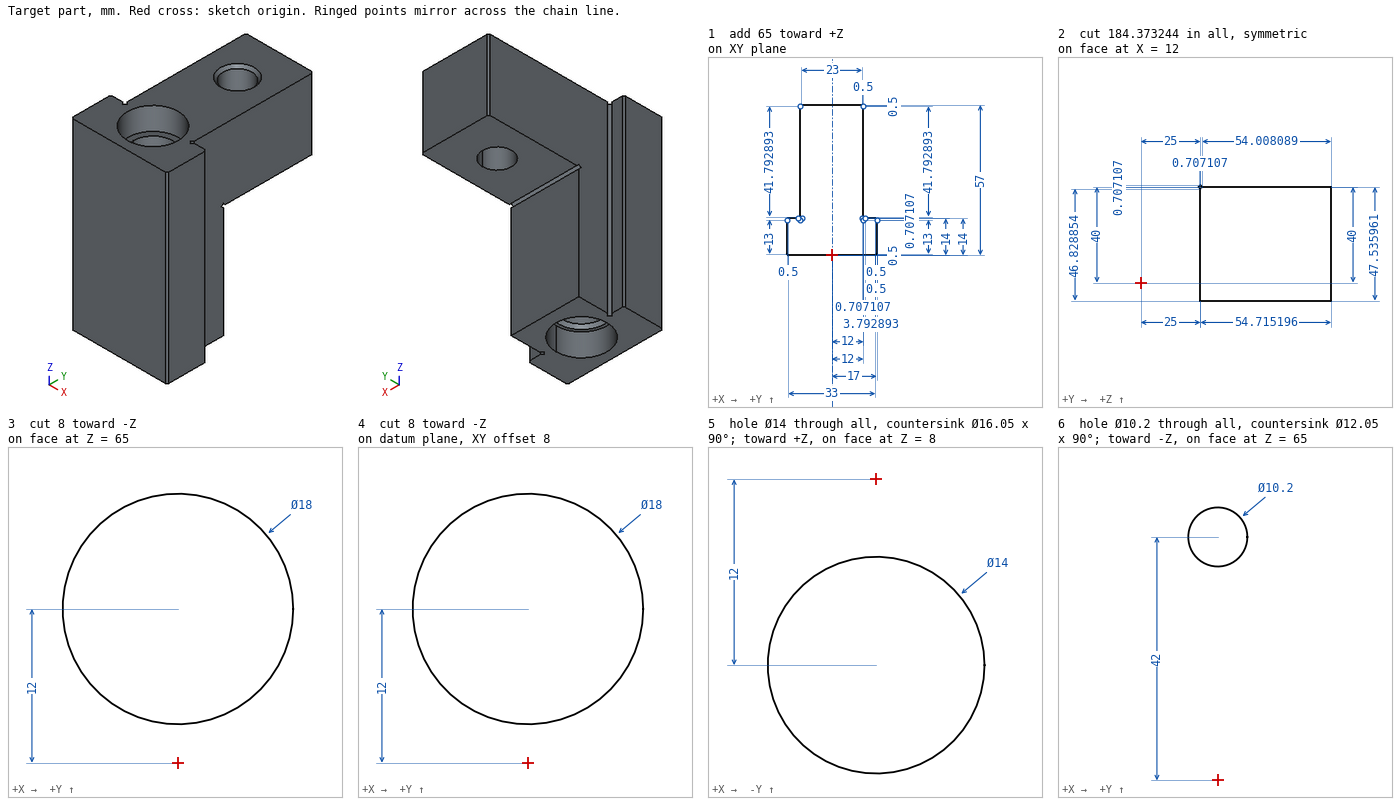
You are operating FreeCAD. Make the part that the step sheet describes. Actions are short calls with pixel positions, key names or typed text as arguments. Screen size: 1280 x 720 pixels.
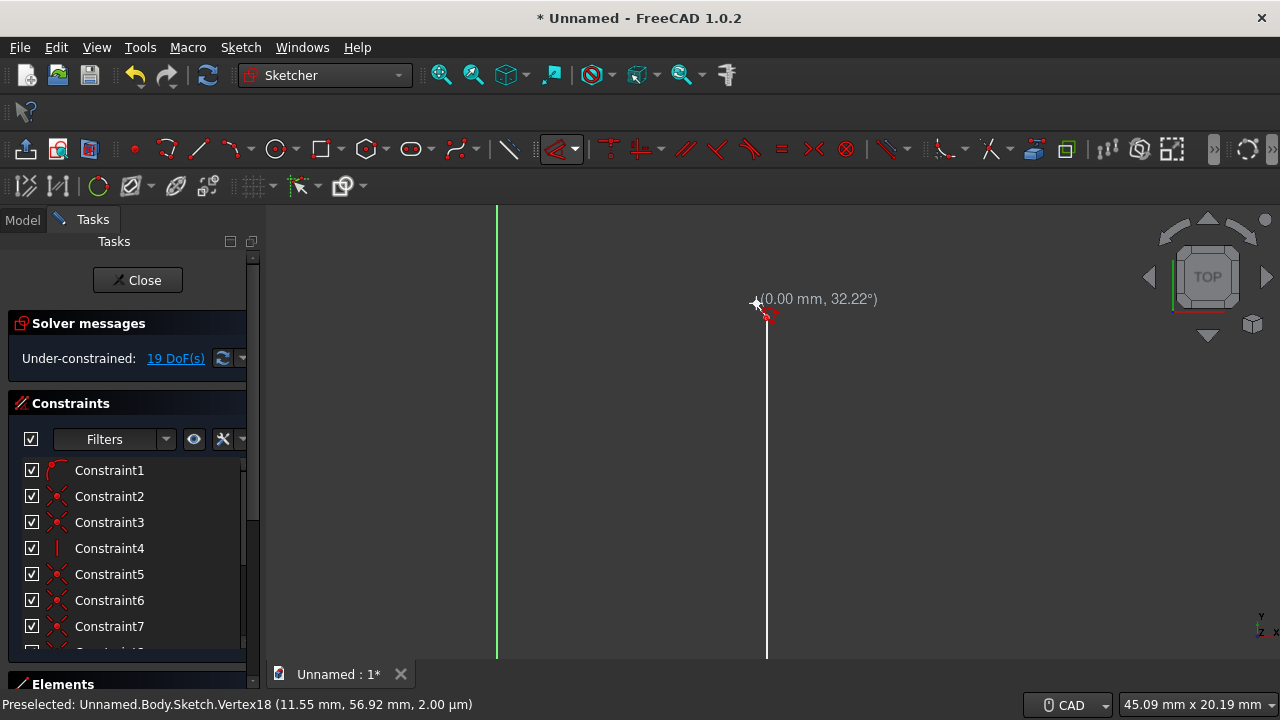
scroll(757, 302, down, 8)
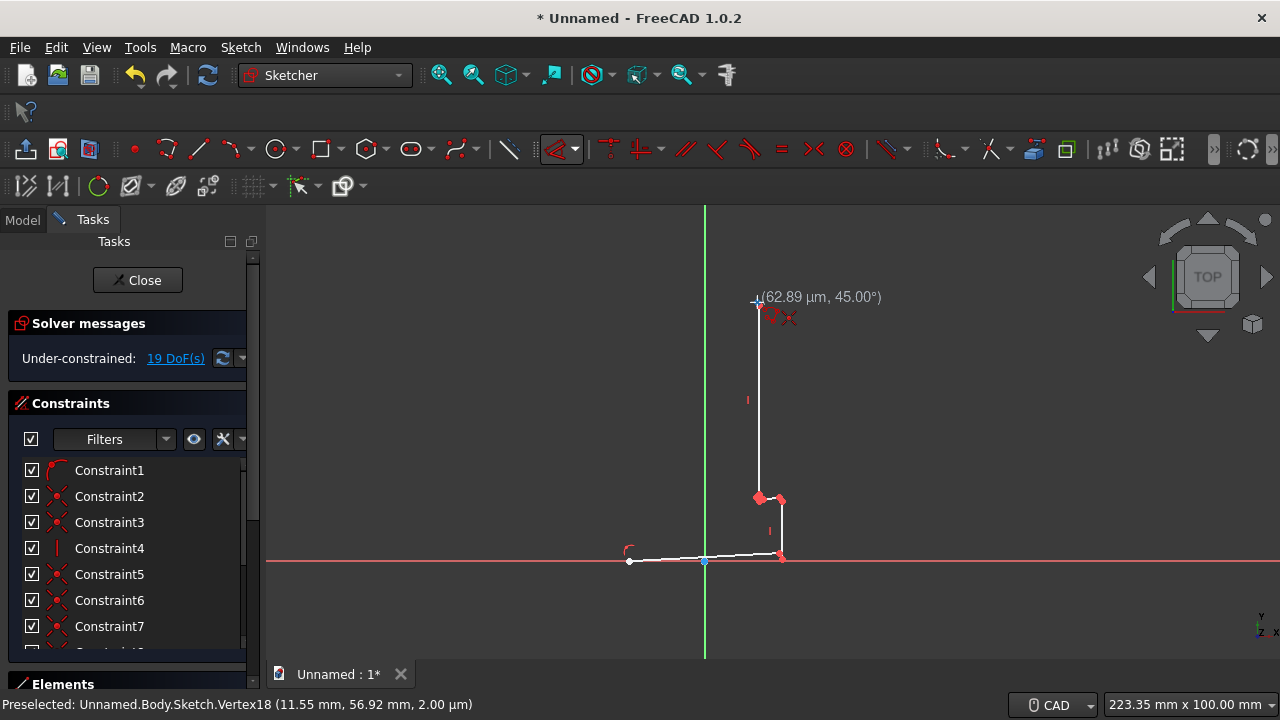
click(653, 302)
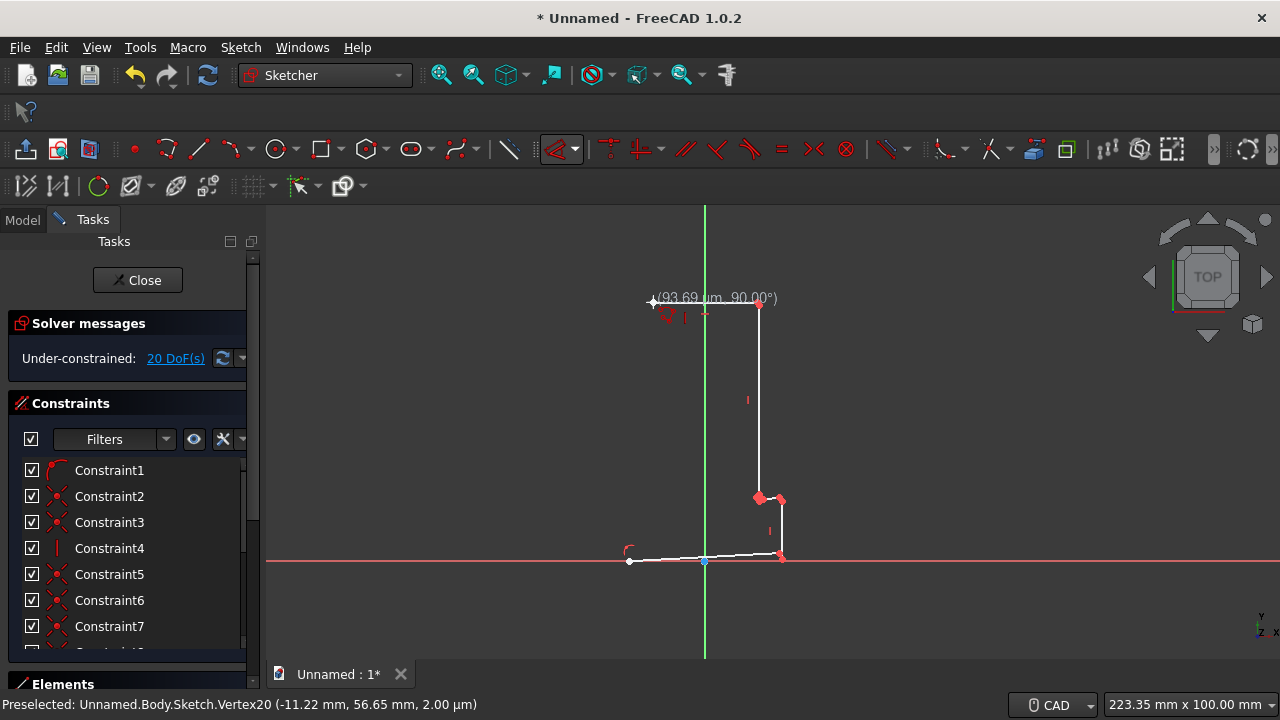
scroll(650, 305, up, 8)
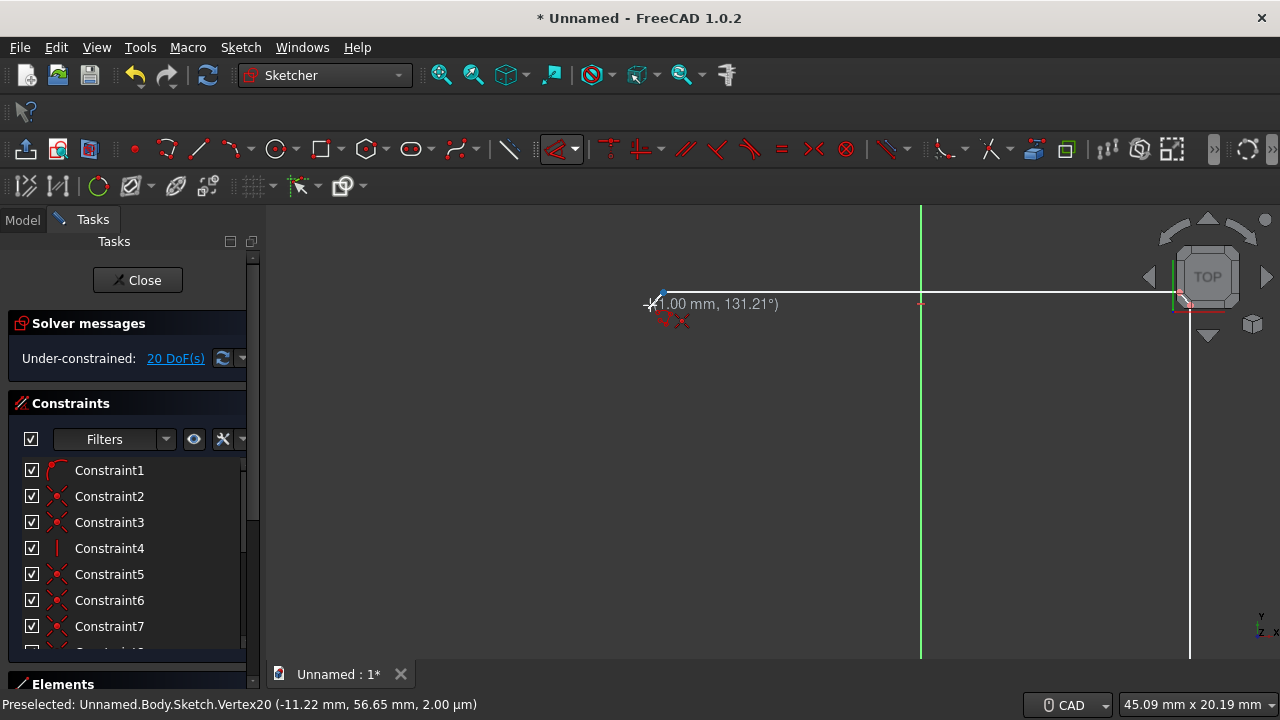
click(651, 303)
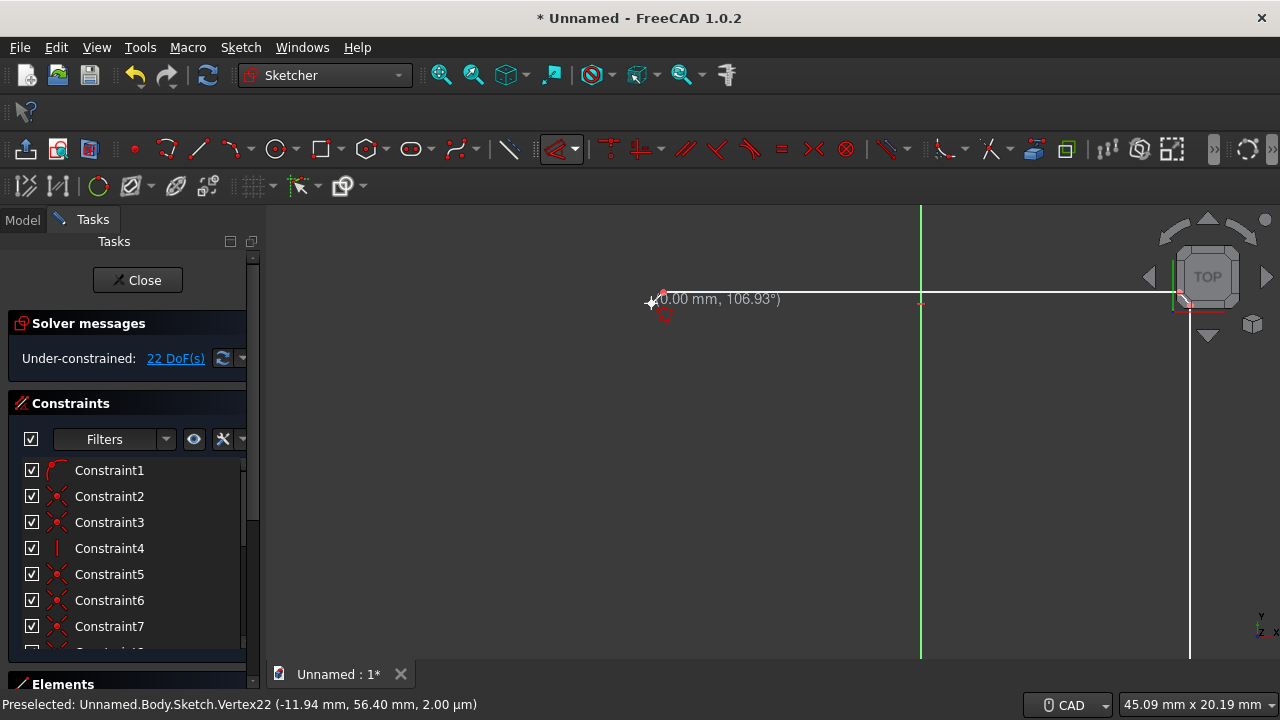
scroll(650, 305, down, 8)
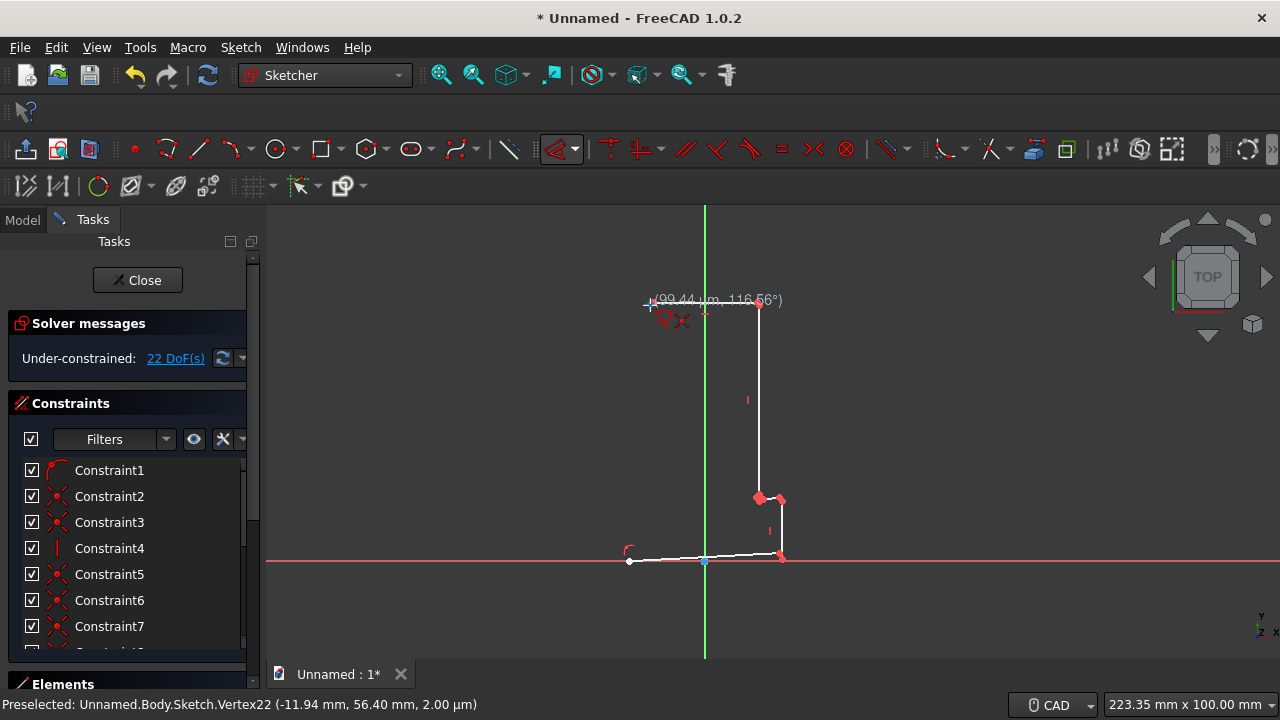
click(651, 494)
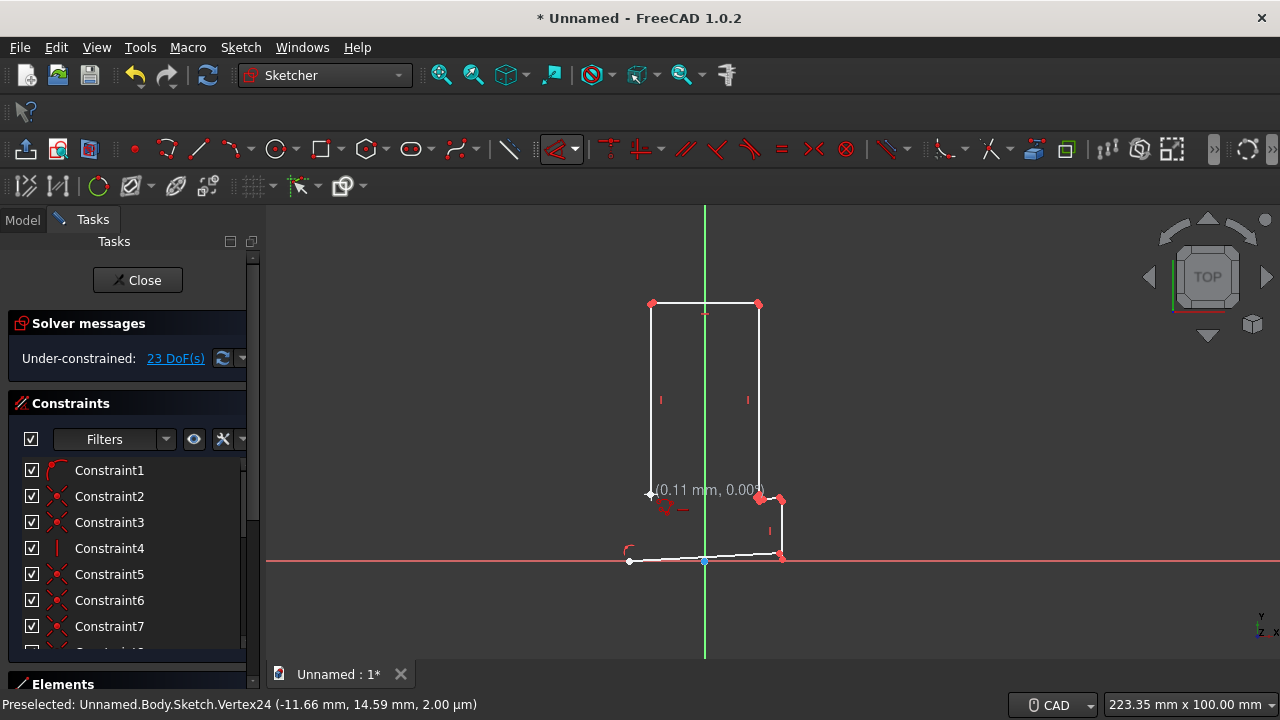
scroll(654, 498, up, 7)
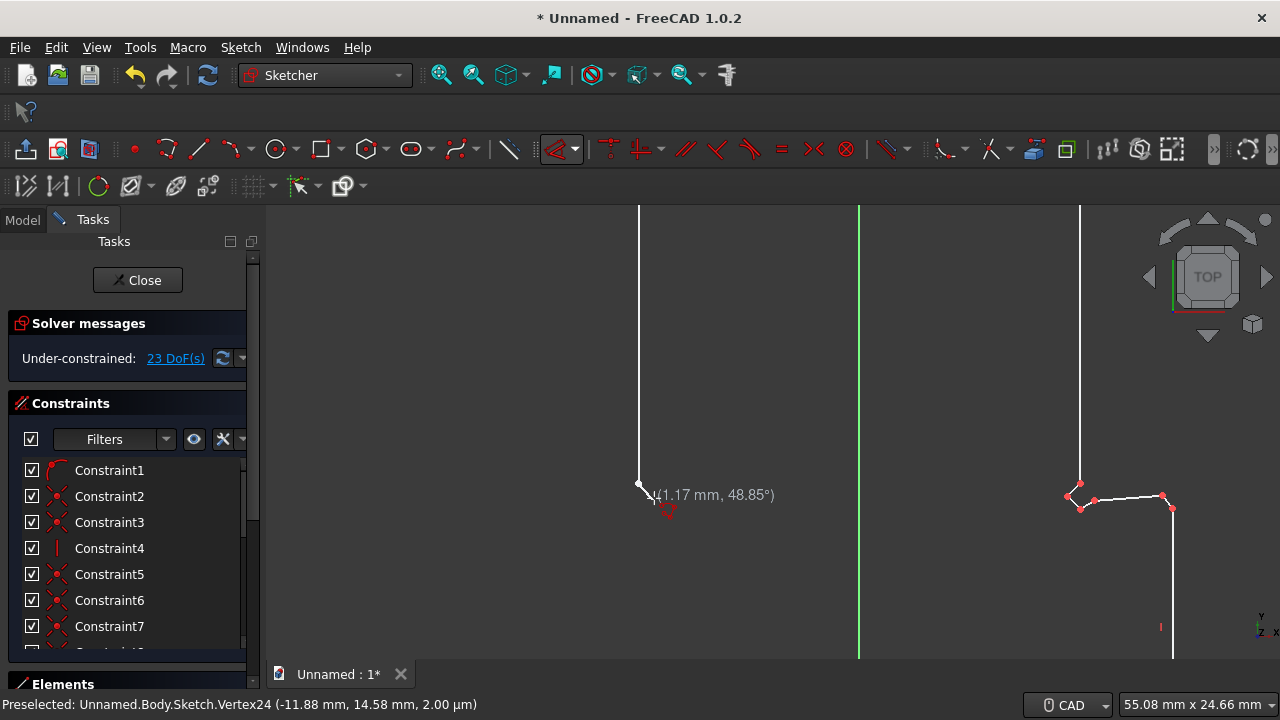
click(652, 495)
click(638, 508)
click(625, 495)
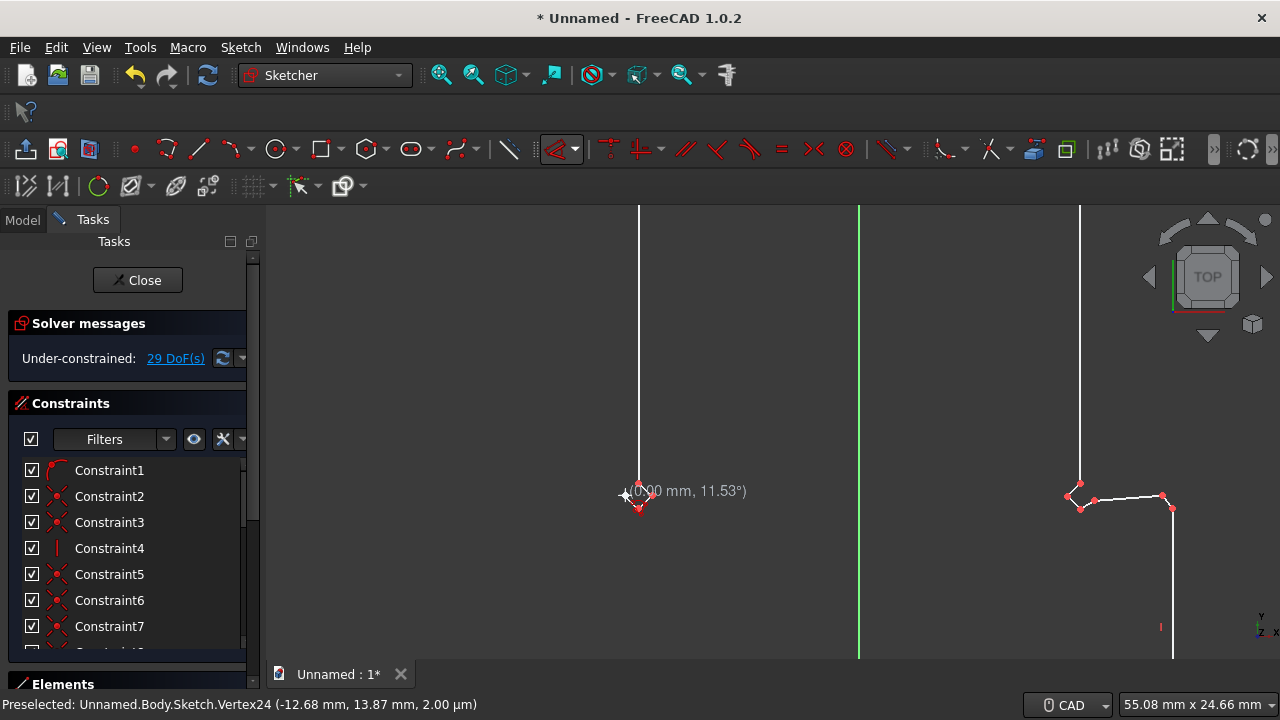
scroll(654, 499, down, 7)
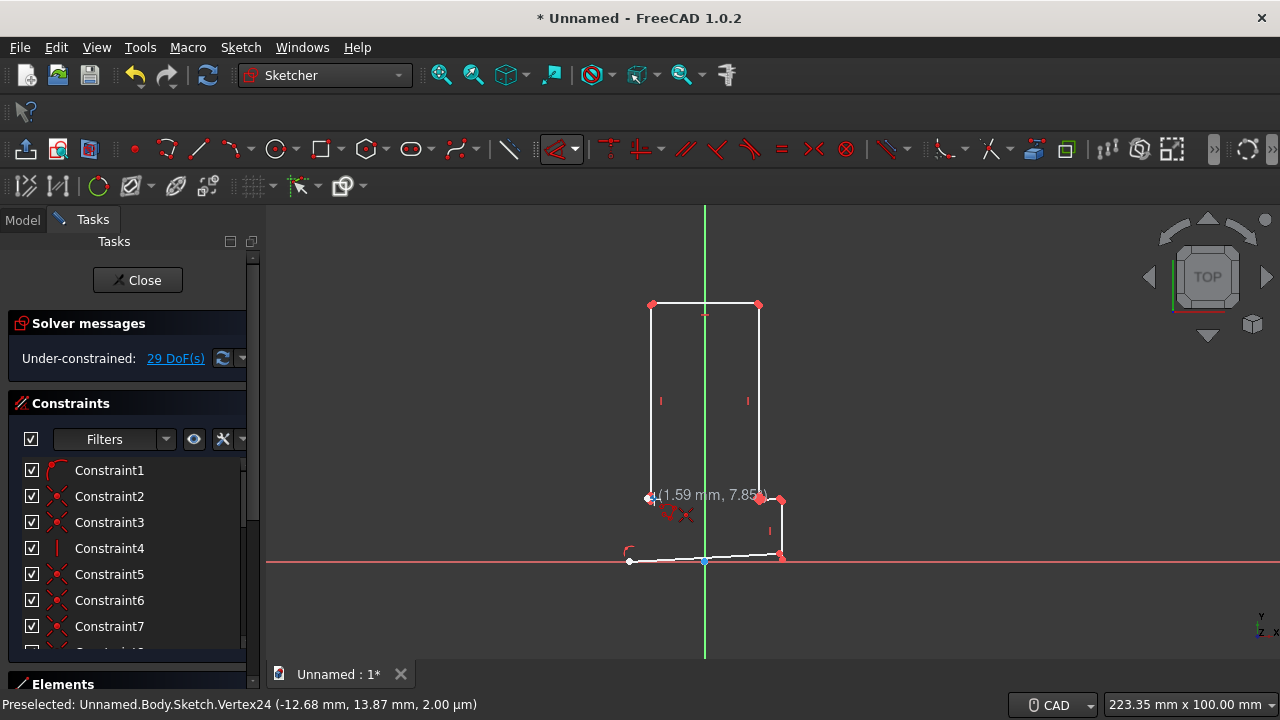
click(630, 499)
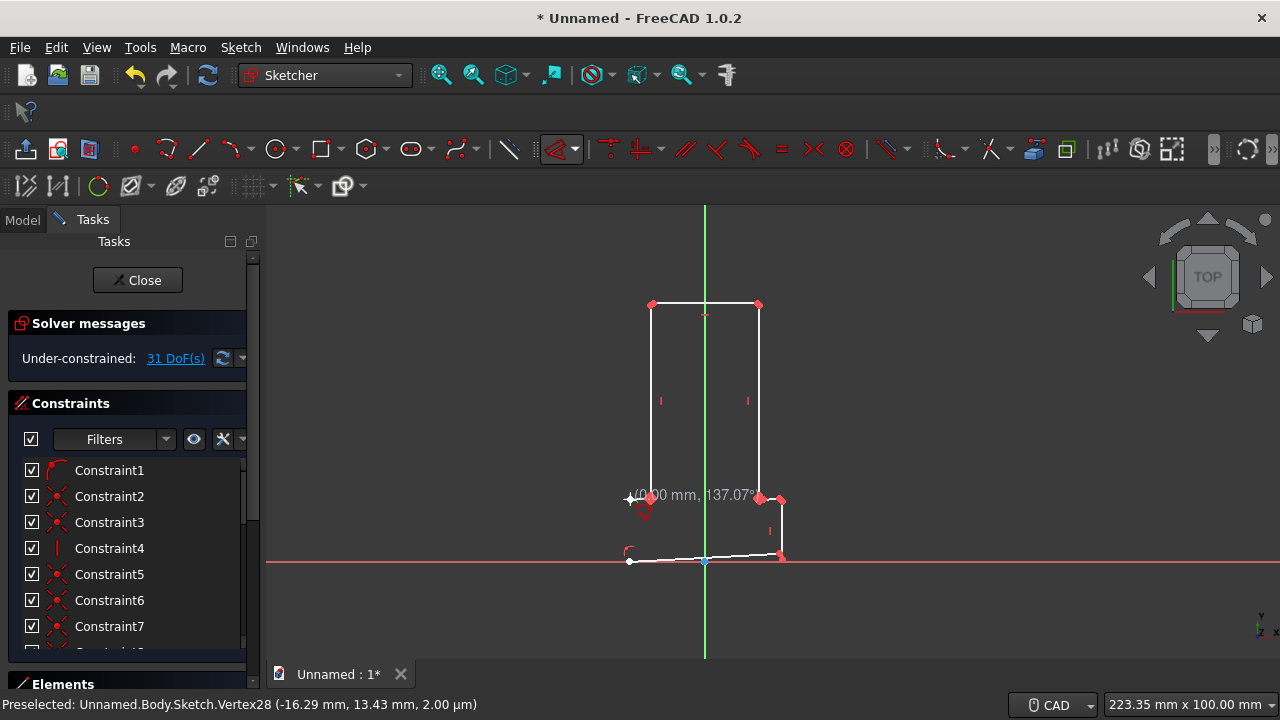
scroll(628, 501, up, 8)